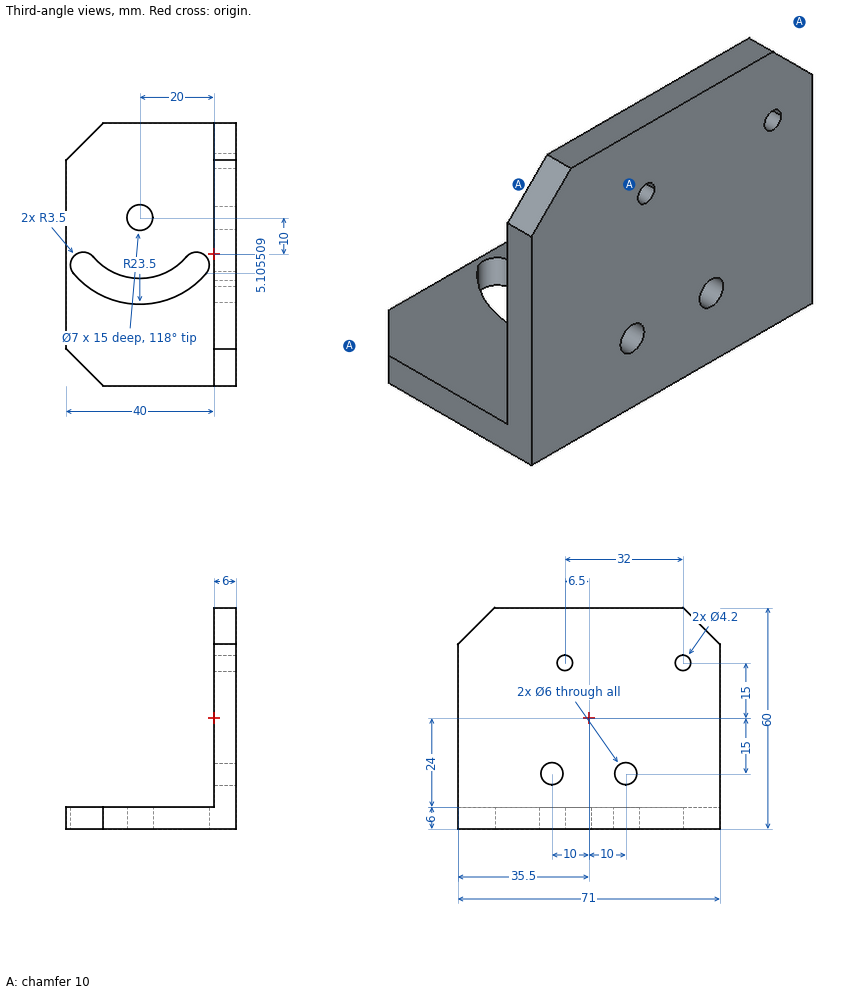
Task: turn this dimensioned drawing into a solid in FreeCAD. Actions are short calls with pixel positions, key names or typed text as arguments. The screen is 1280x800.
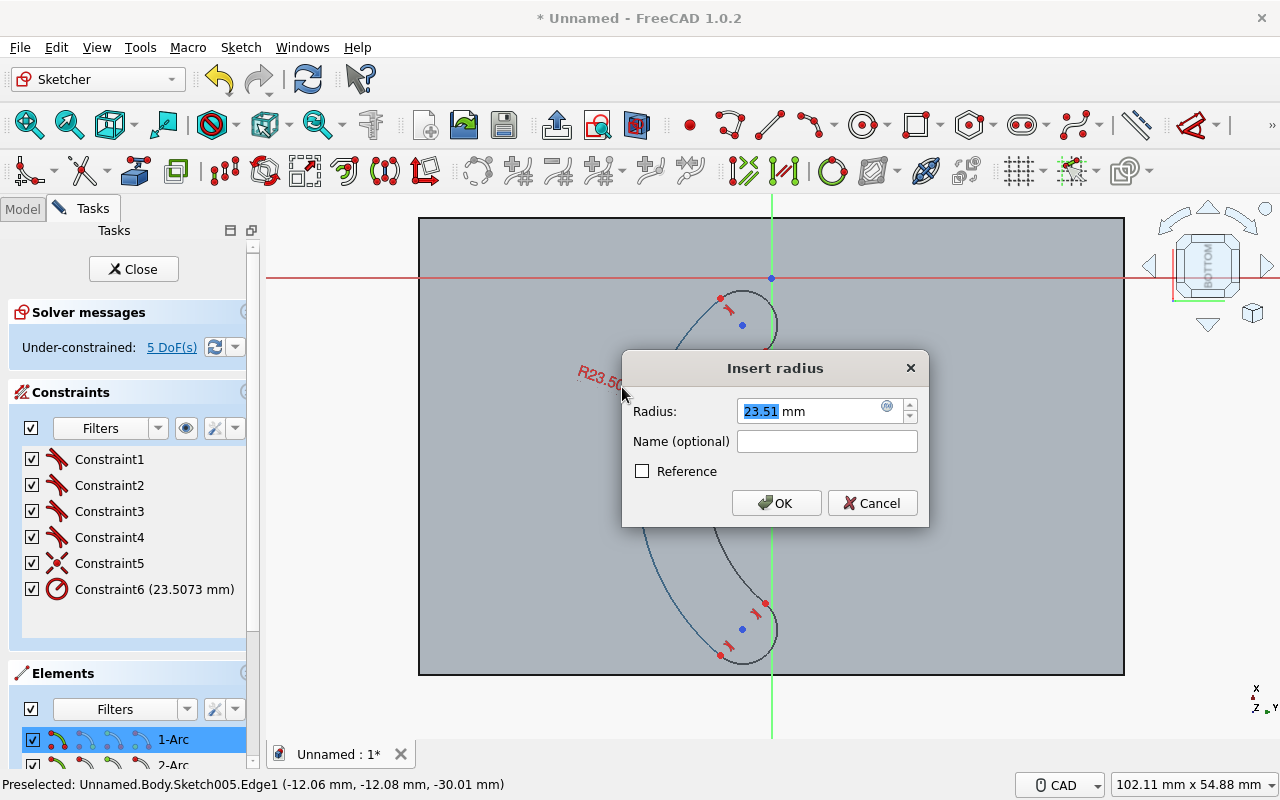
text(23.5)
key(Return)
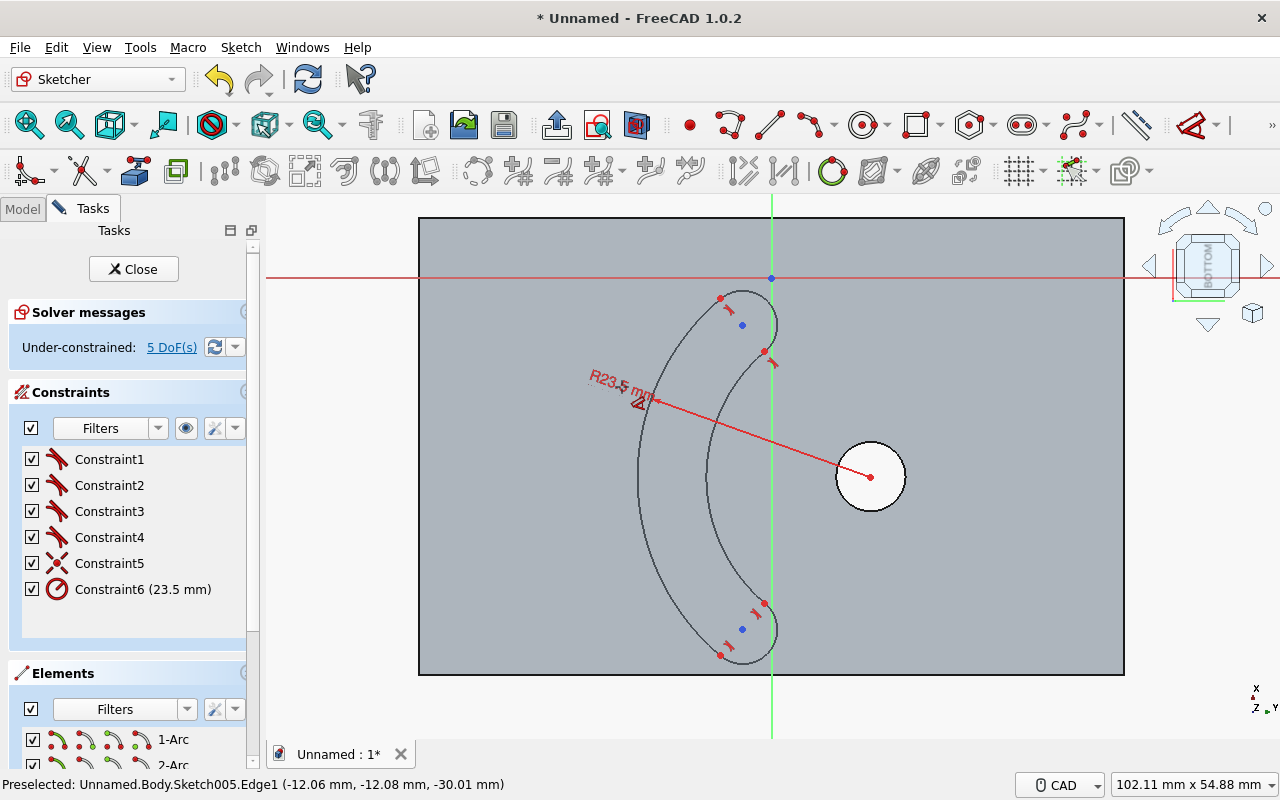
click(751, 663)
click(726, 694)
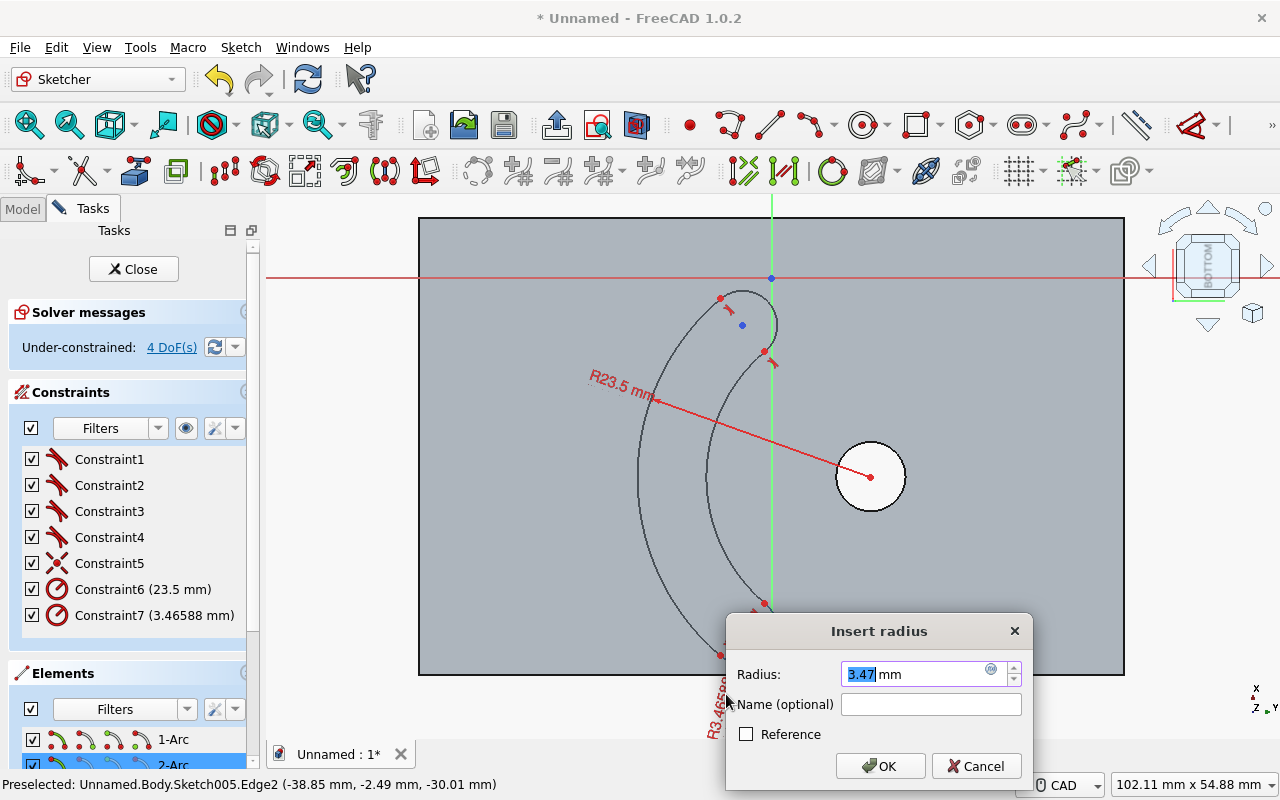
text(3.5)
key(Return)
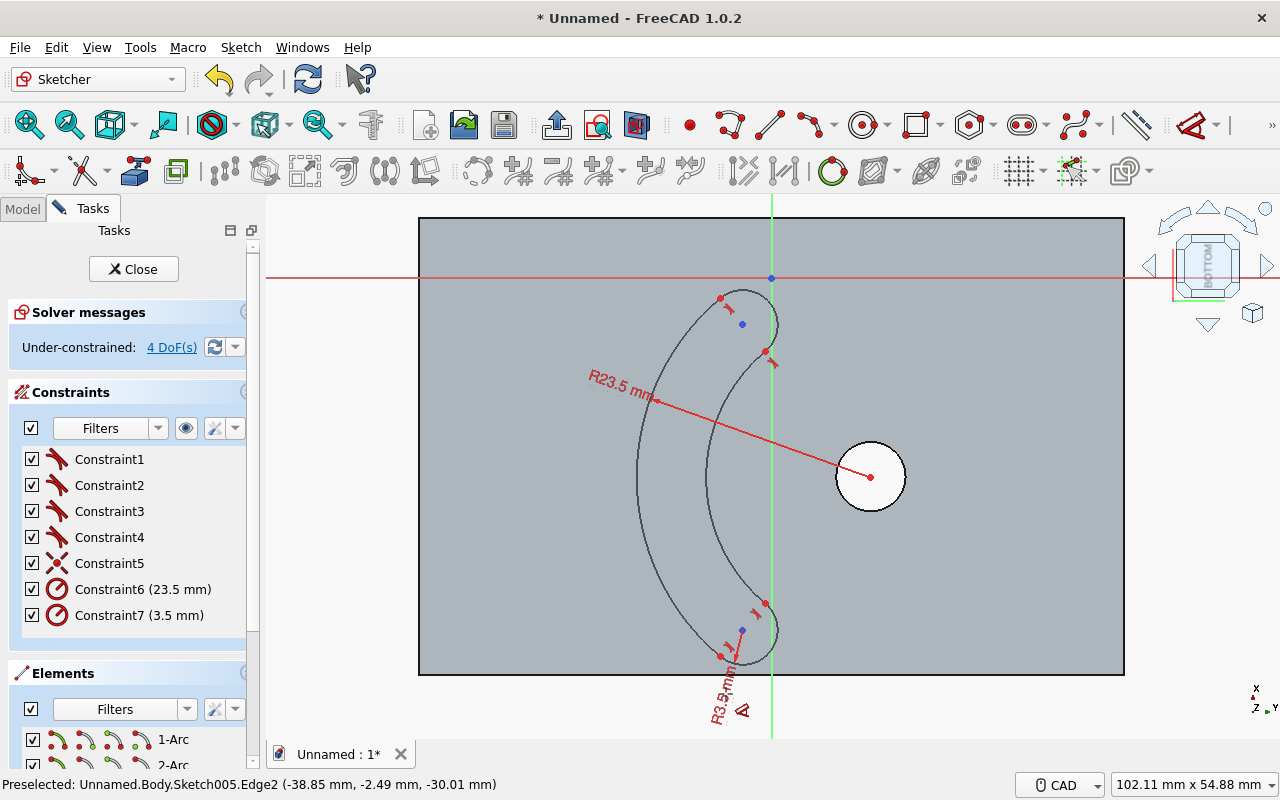
click(870, 477)
click(821, 244)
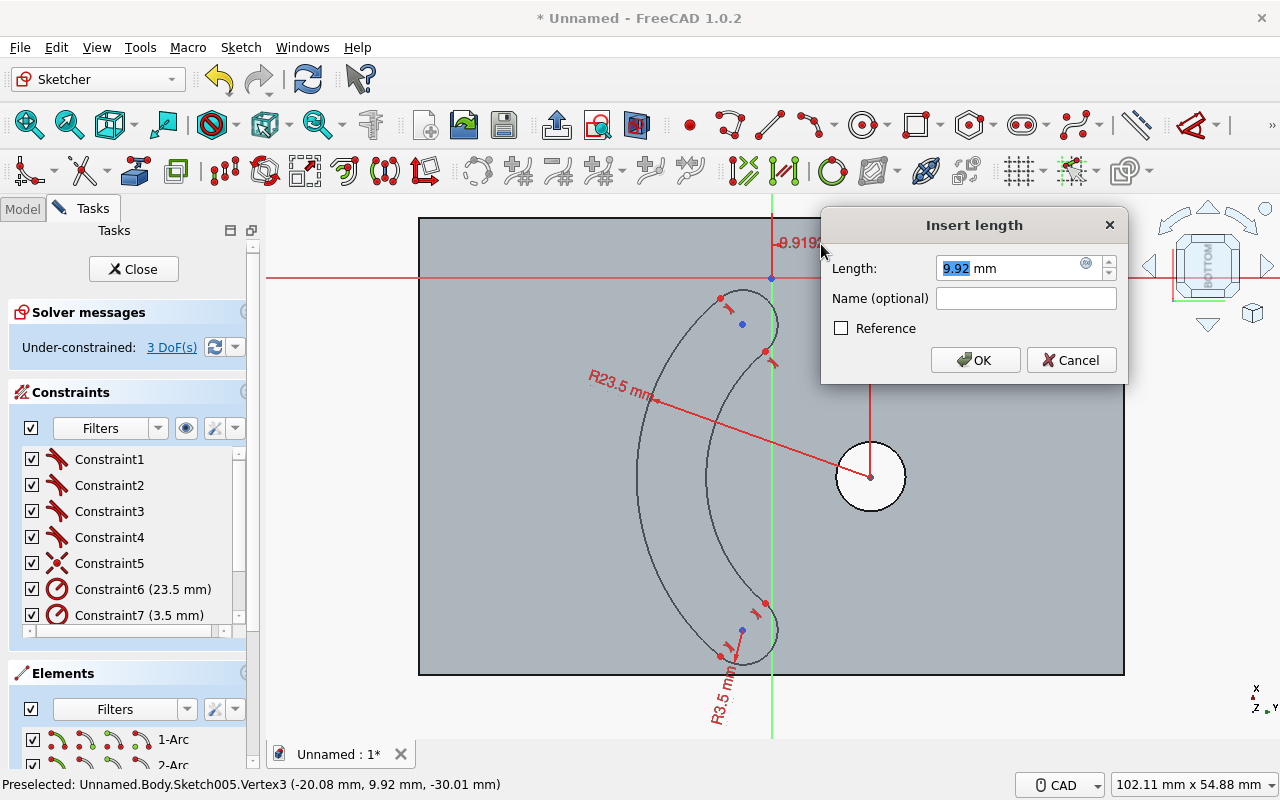
text(10)
key(Return)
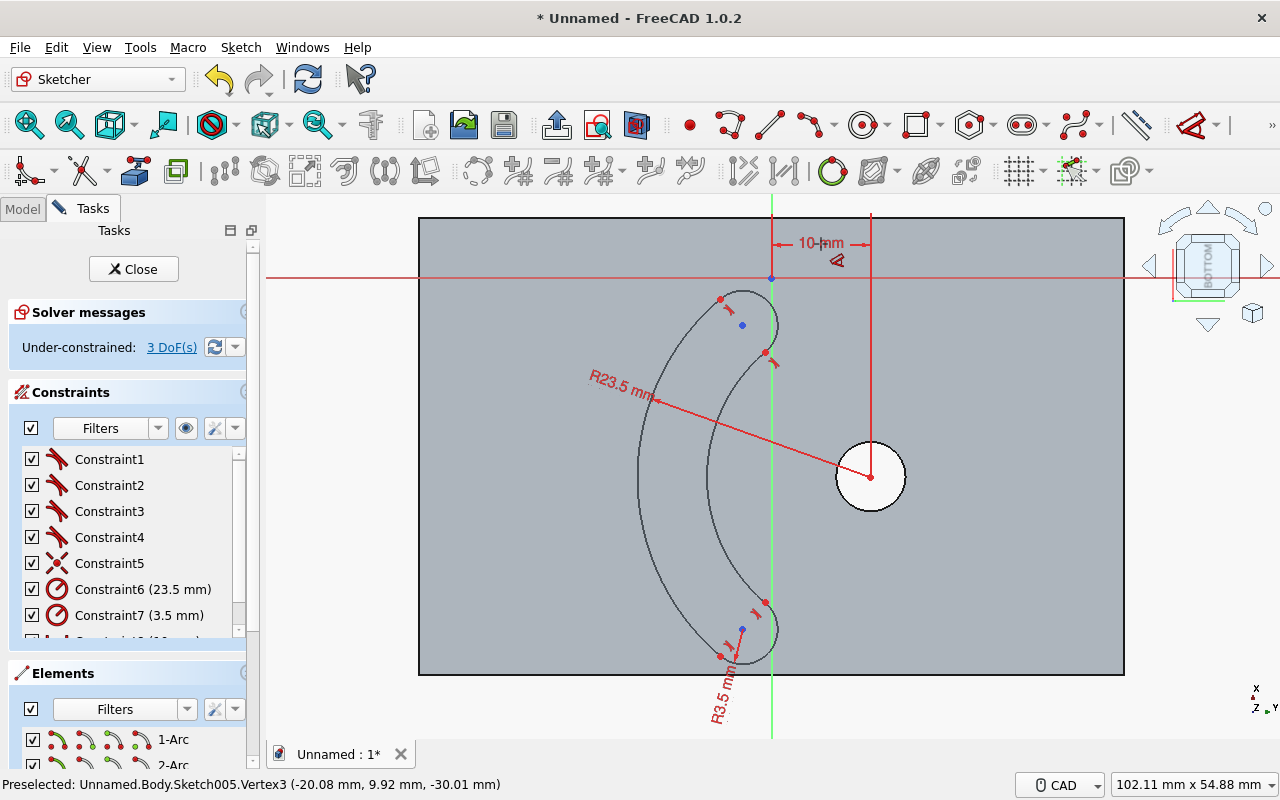
click(871, 478)
click(905, 378)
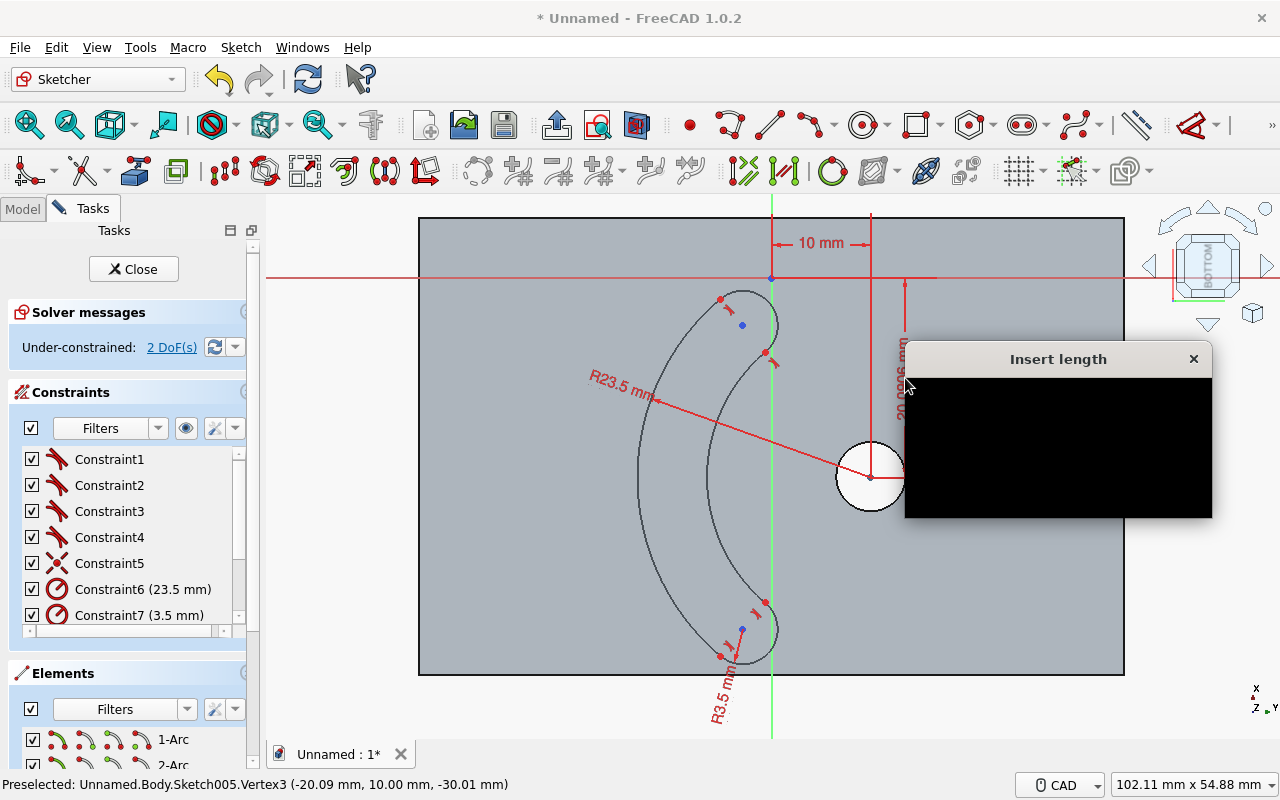
text(20)
key(Return)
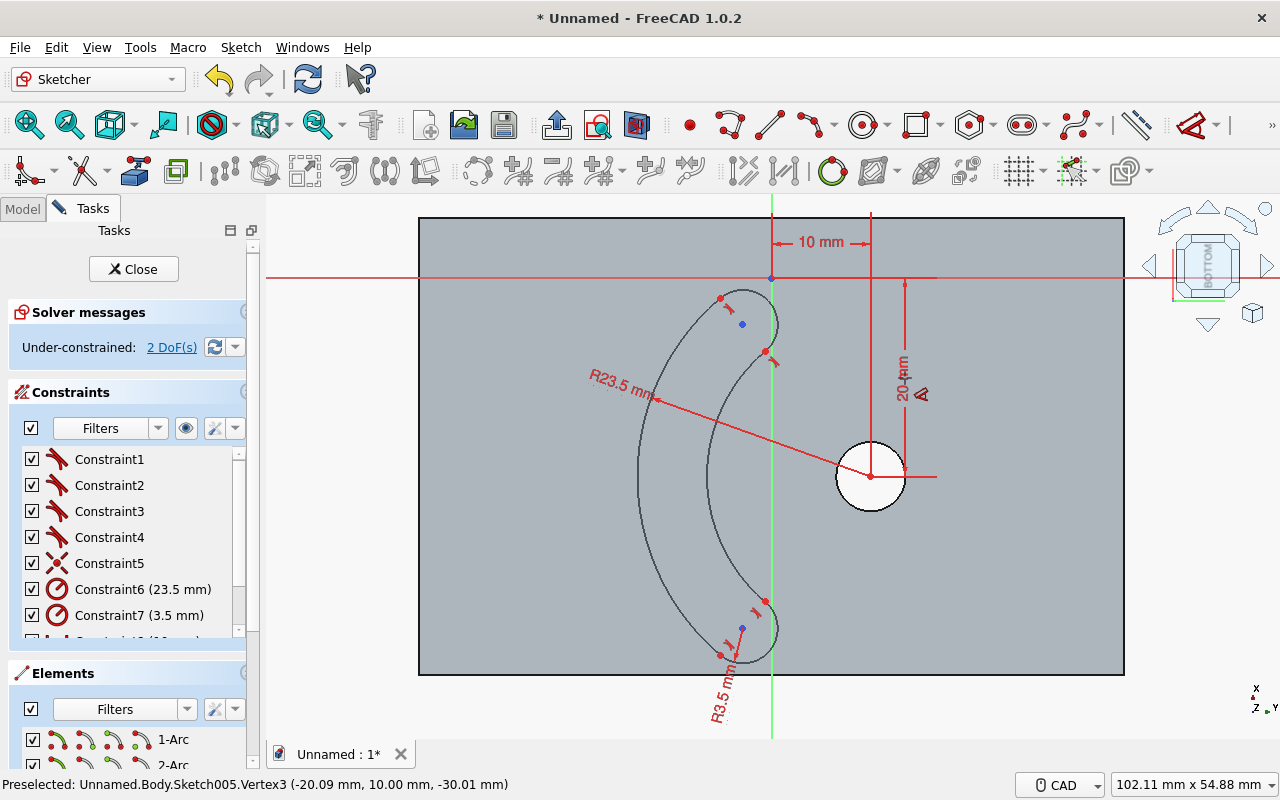
click(721, 298)
click(746, 244)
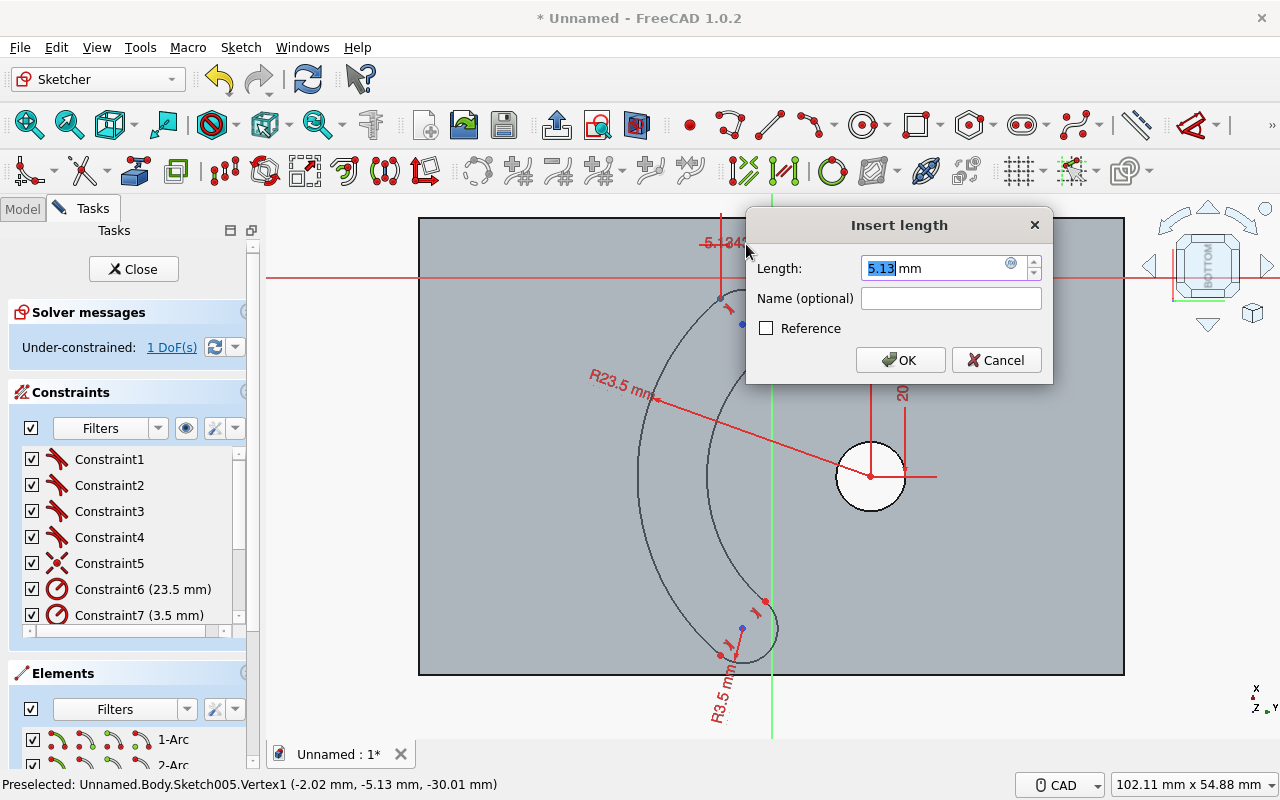
text(5.105509)
key(Return)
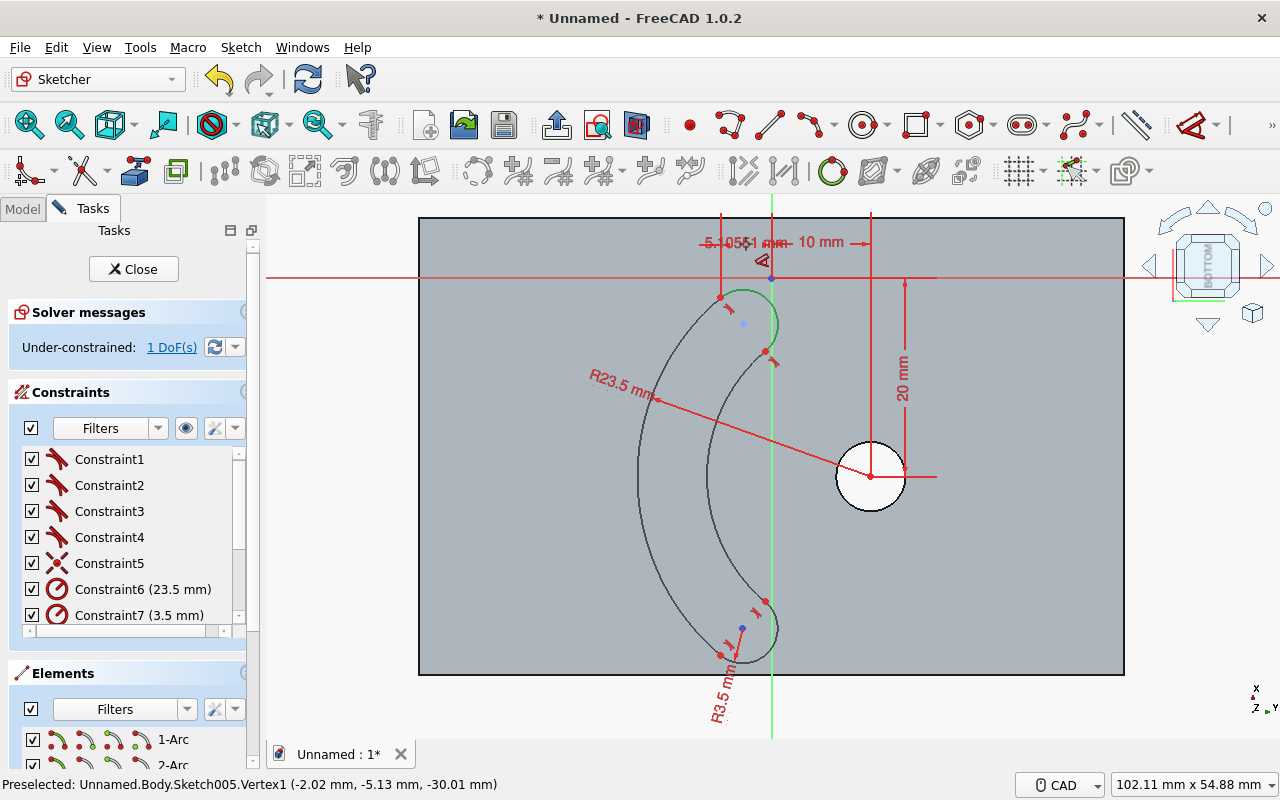
click(721, 655)
click(764, 689)